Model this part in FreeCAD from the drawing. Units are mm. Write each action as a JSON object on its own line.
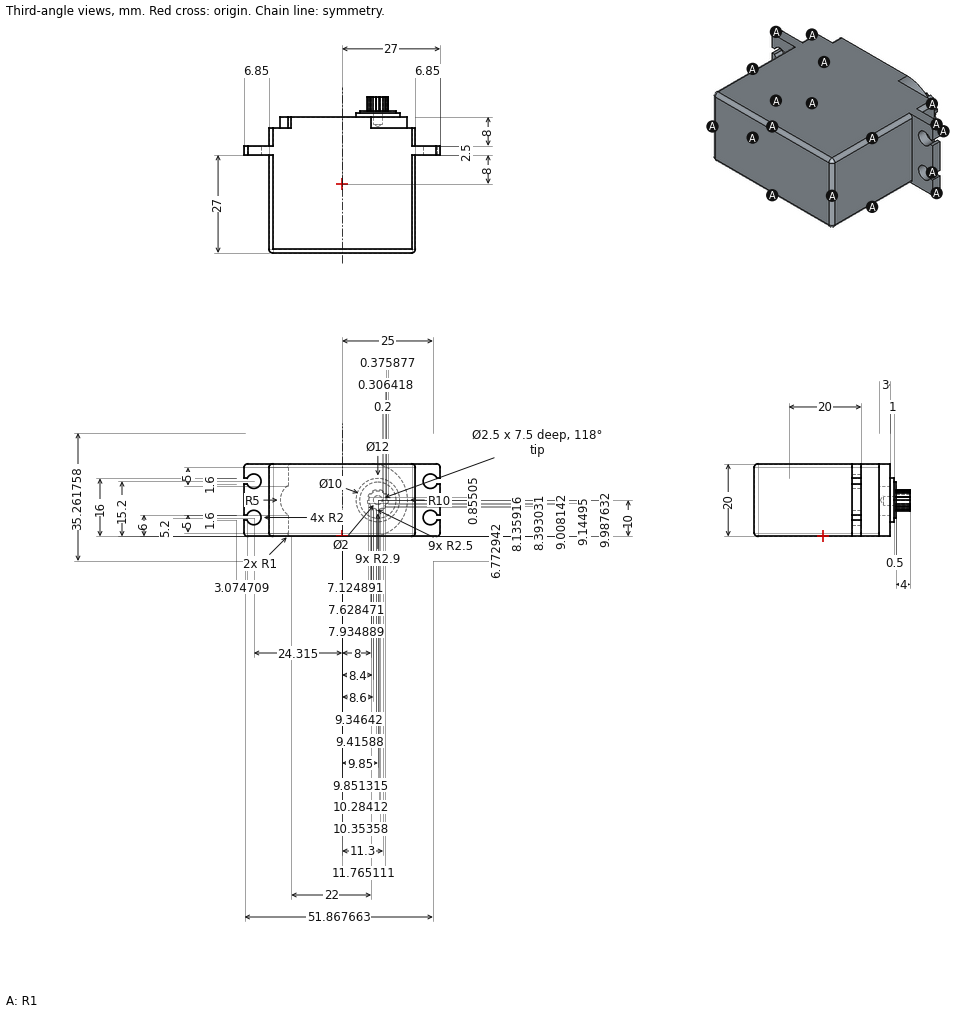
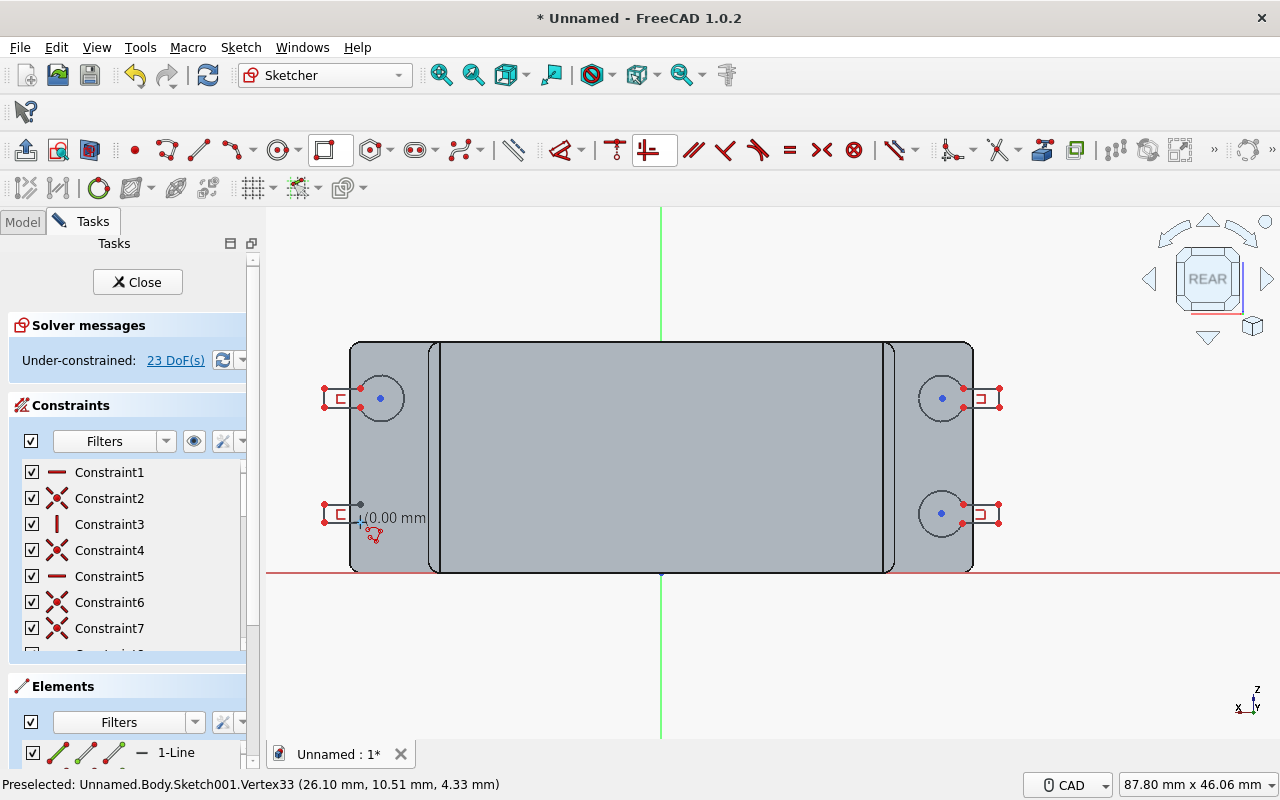
{"action": "left_click", "coordinate": [232, 150]}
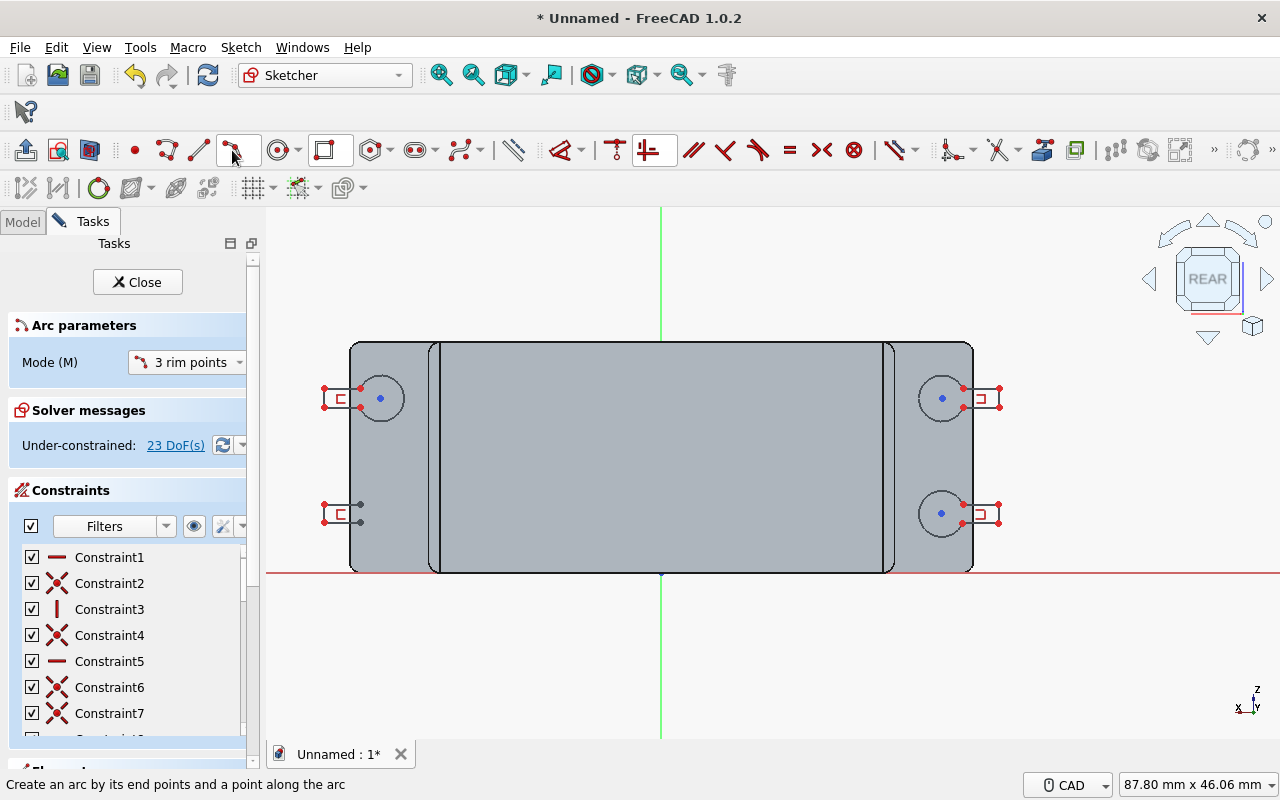
{"action": "left_click", "coordinate": [360, 523]}
{"action": "left_click", "coordinate": [360, 505]}
{"action": "left_click", "coordinate": [404, 513]}
{"action": "key", "text": "Escape"}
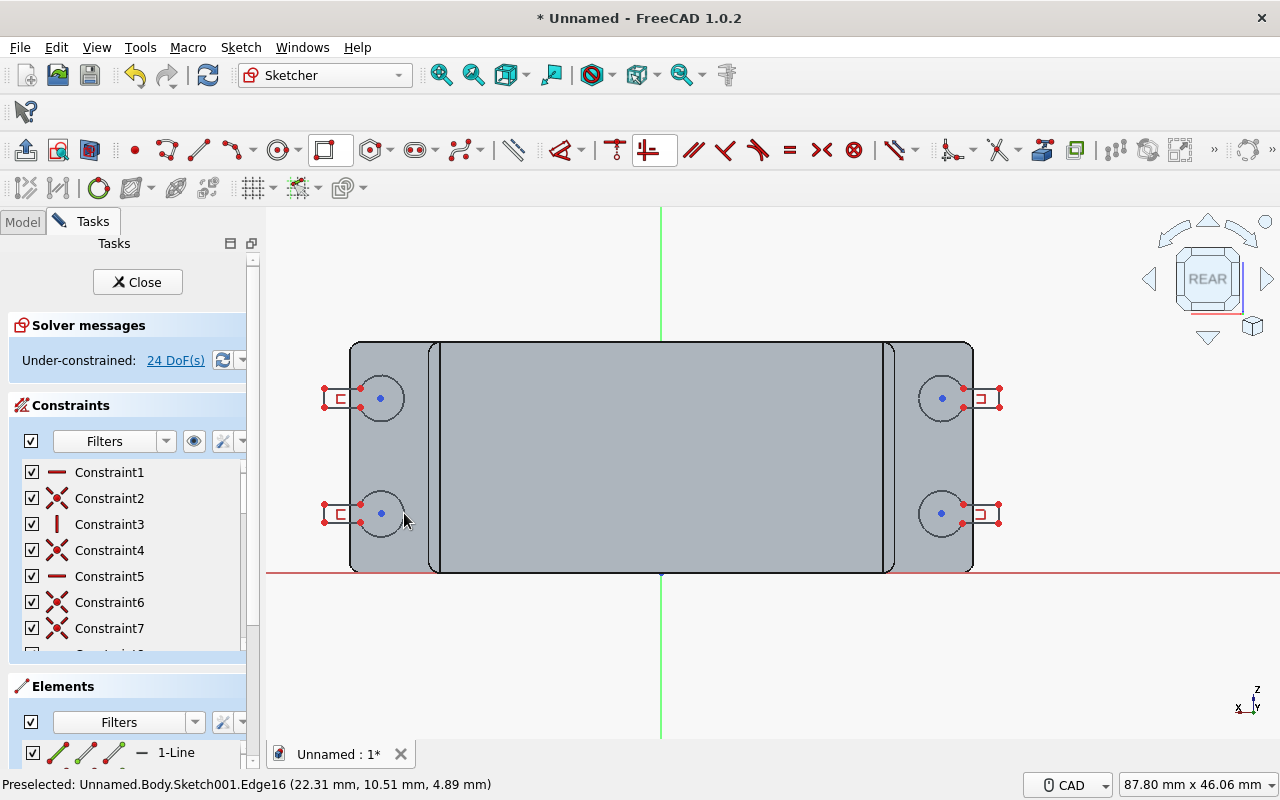
{"action": "left_click", "coordinate": [932, 493]}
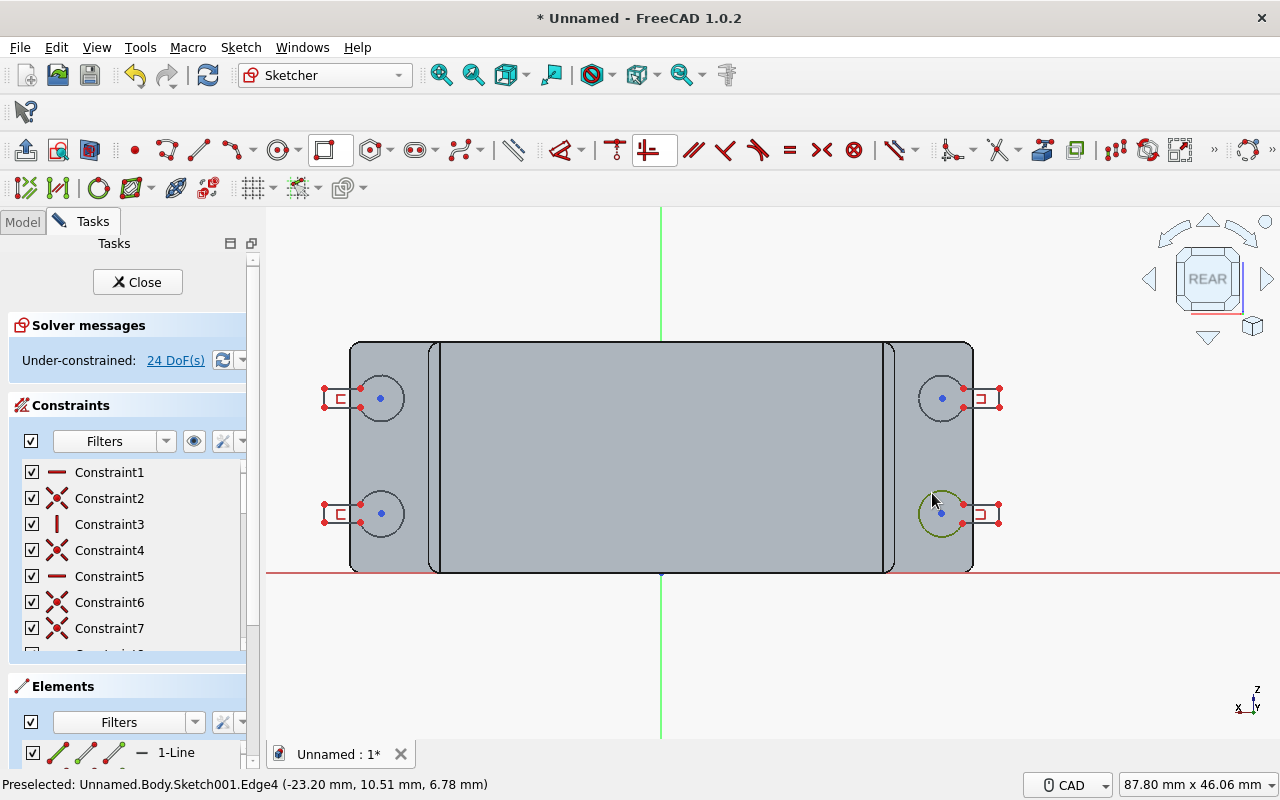
{"action": "left_click", "coordinate": [931, 378]}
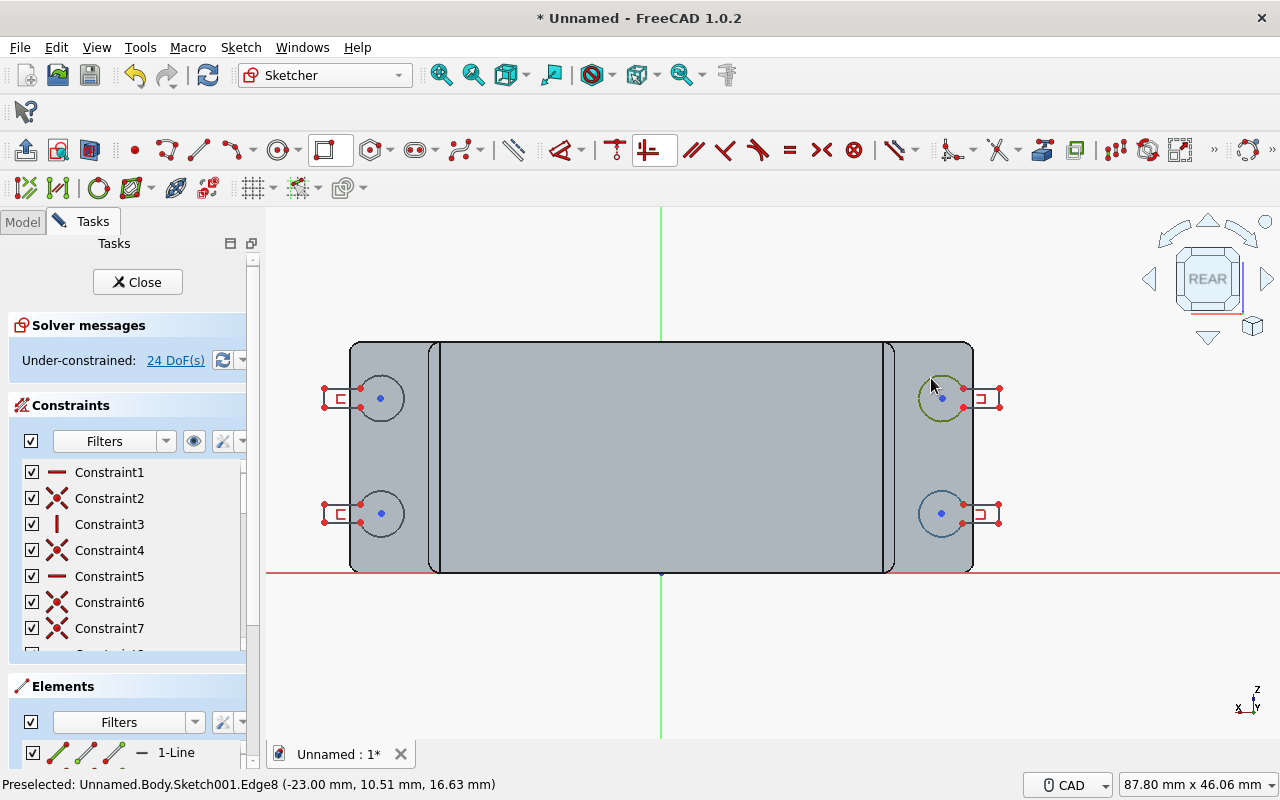
{"action": "left_click", "coordinate": [392, 419]}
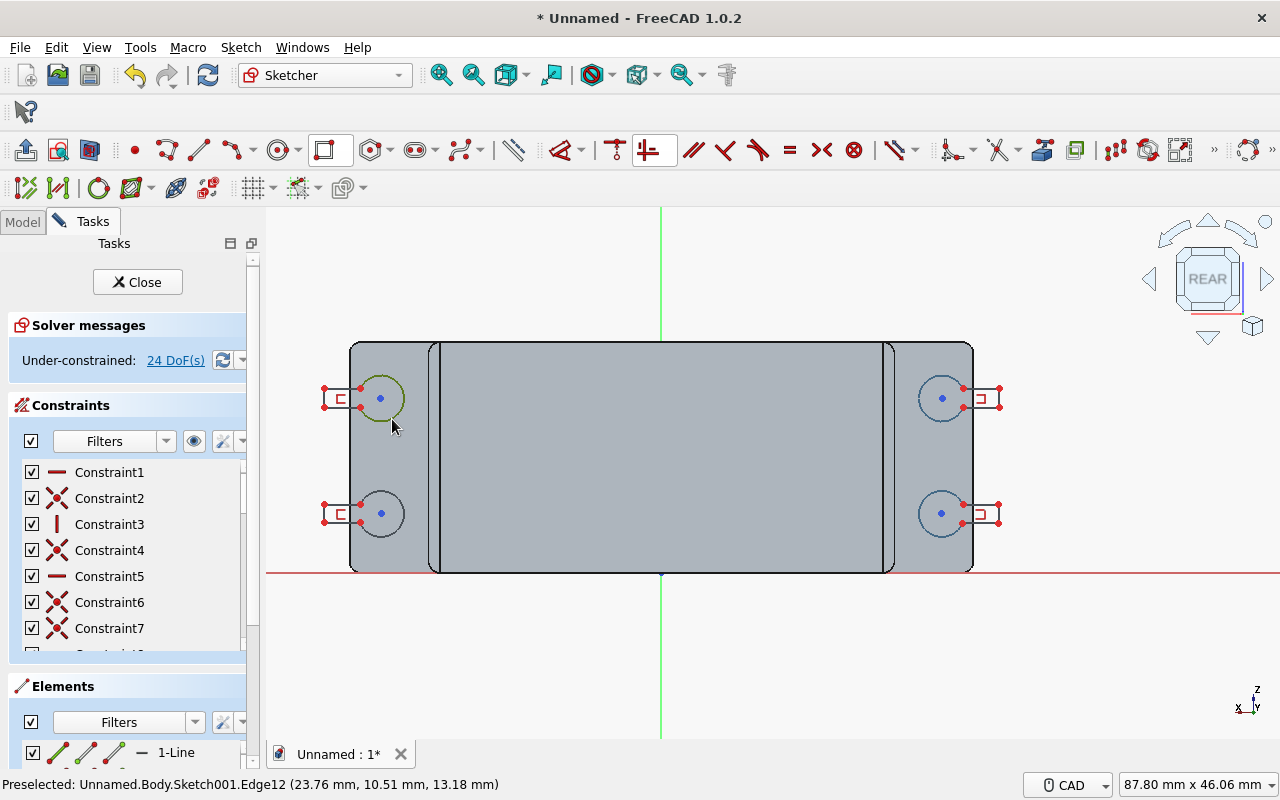
{"action": "left_click", "coordinate": [392, 534]}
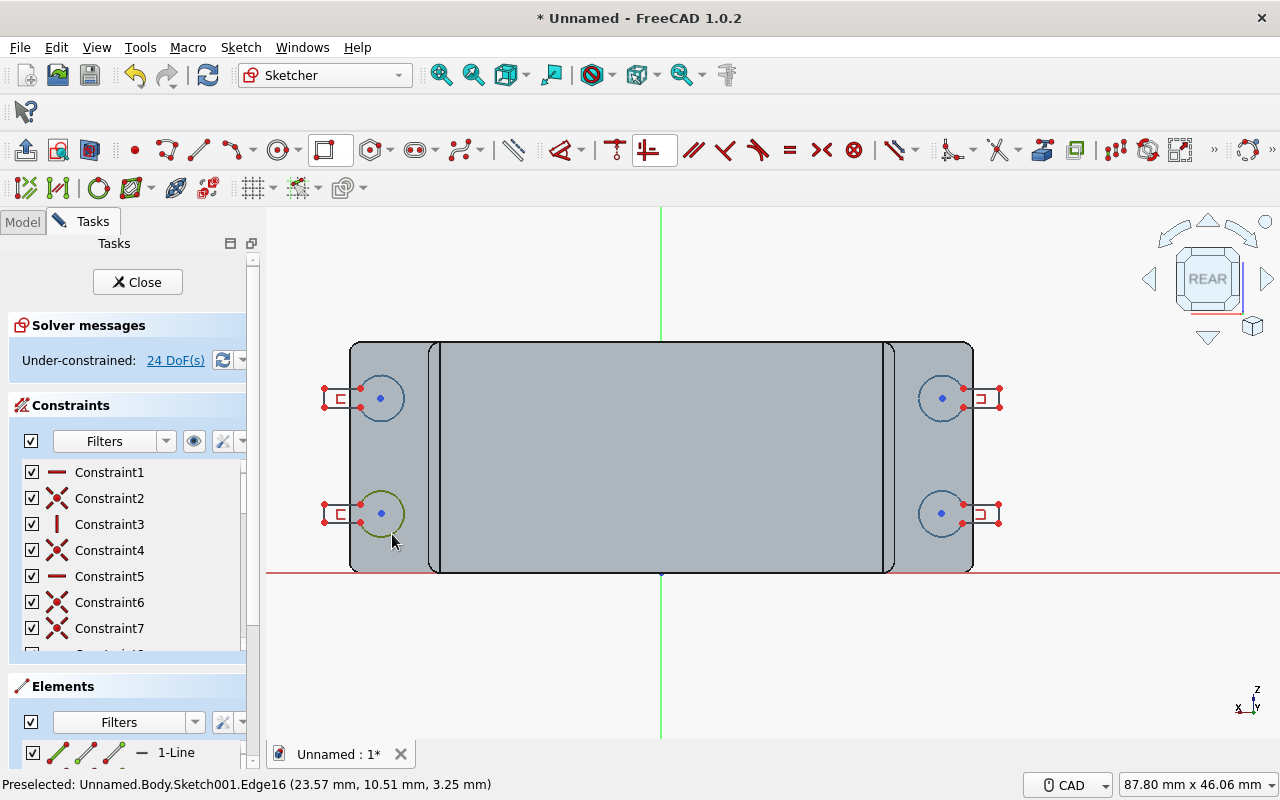
{"action": "left_click", "coordinate": [790, 150]}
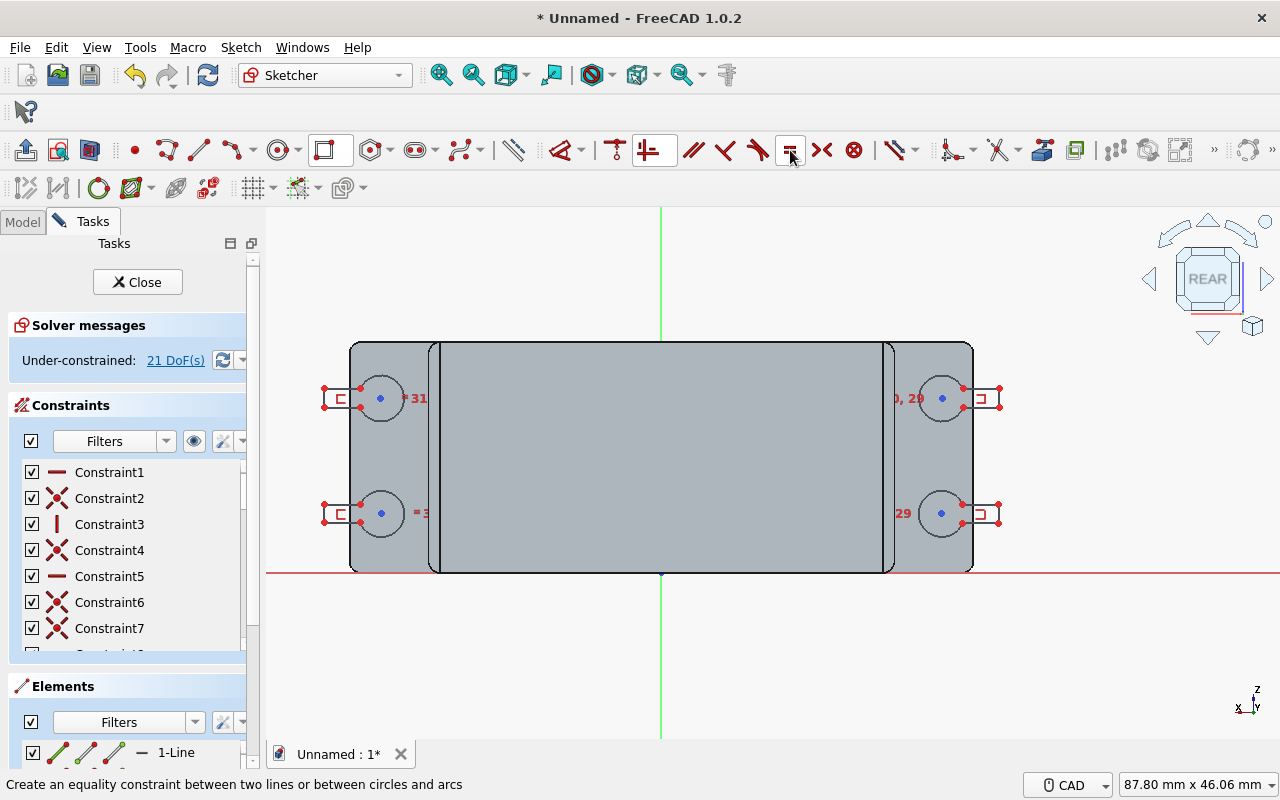
{"action": "left_click", "coordinate": [942, 399]}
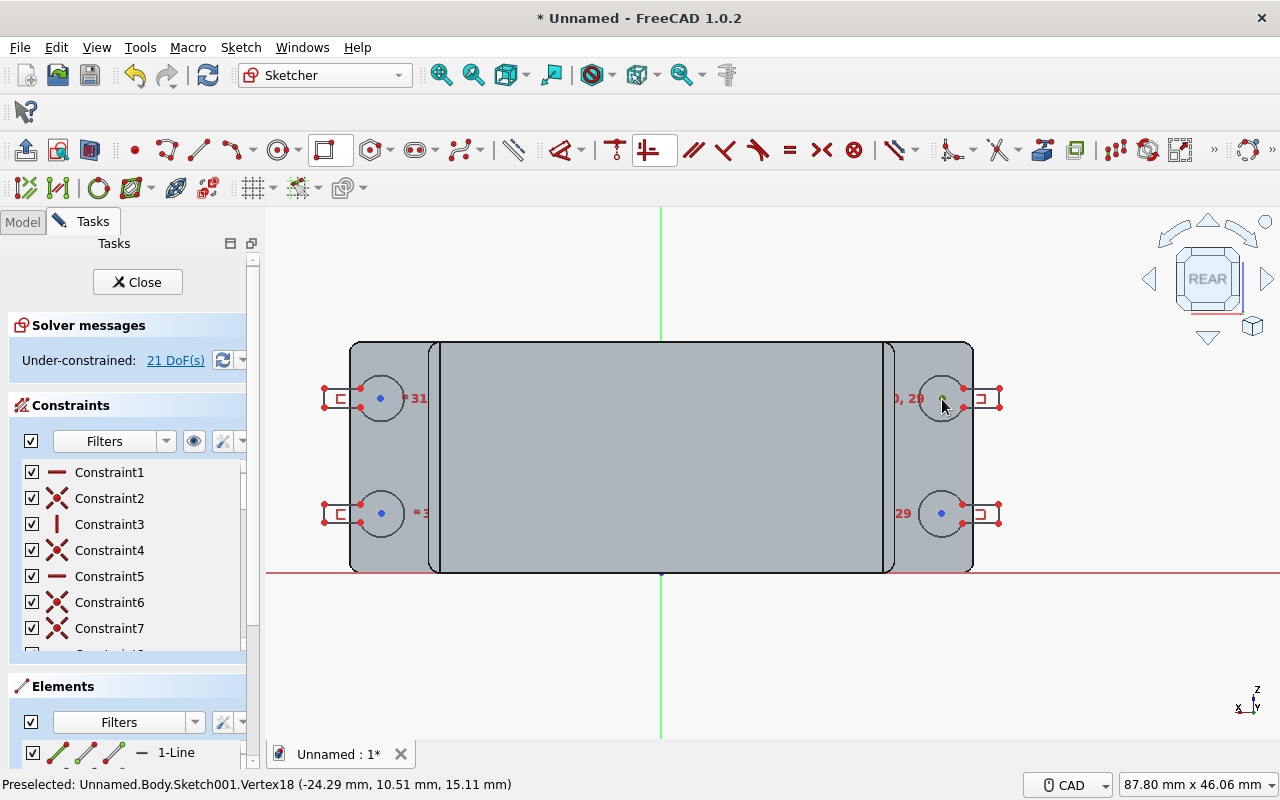
{"action": "left_click", "coordinate": [381, 399]}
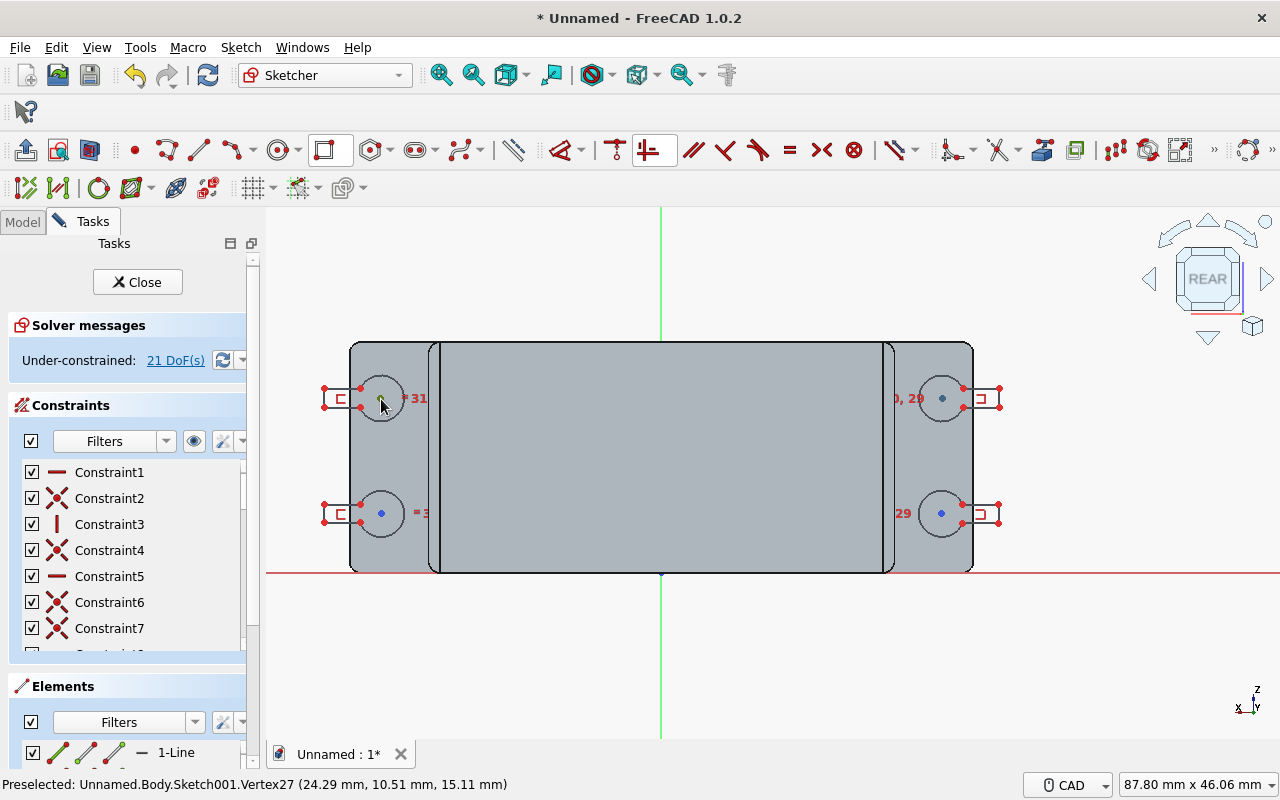
{"action": "left_click", "coordinate": [661, 677]}